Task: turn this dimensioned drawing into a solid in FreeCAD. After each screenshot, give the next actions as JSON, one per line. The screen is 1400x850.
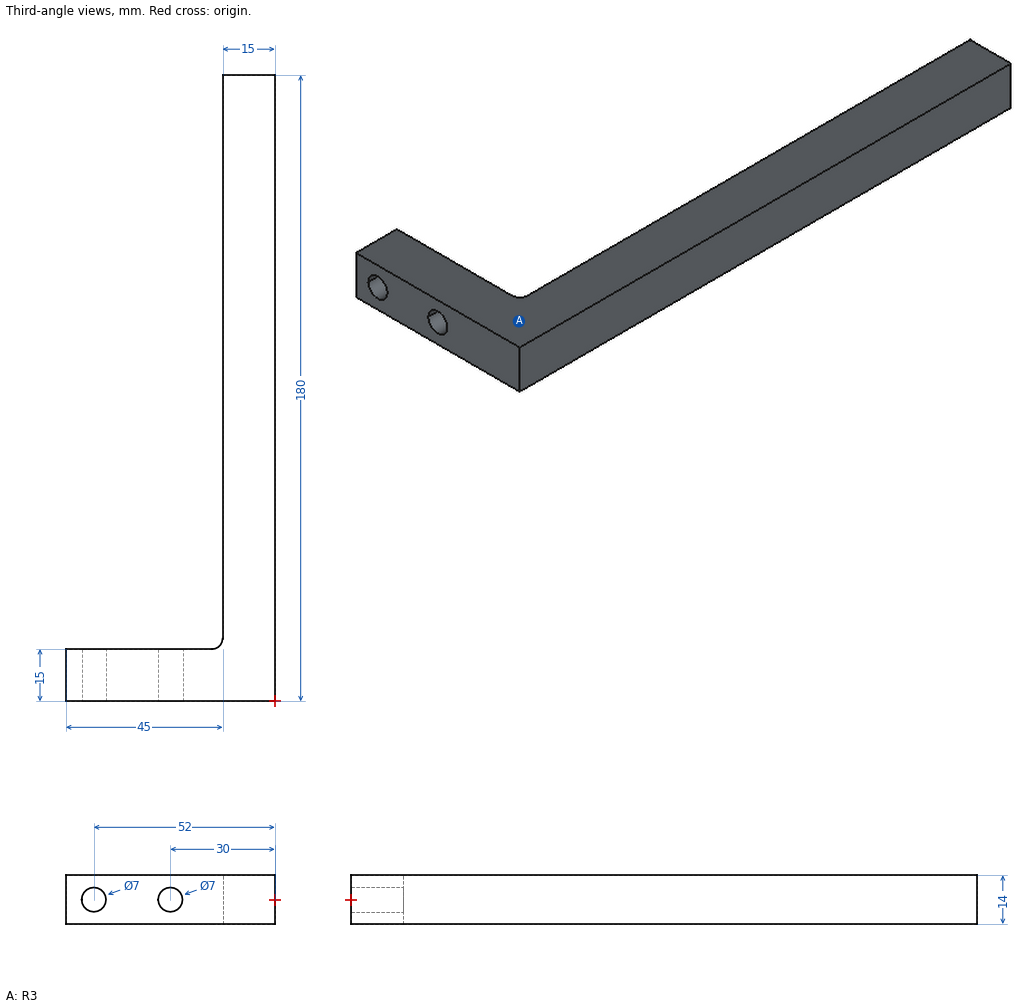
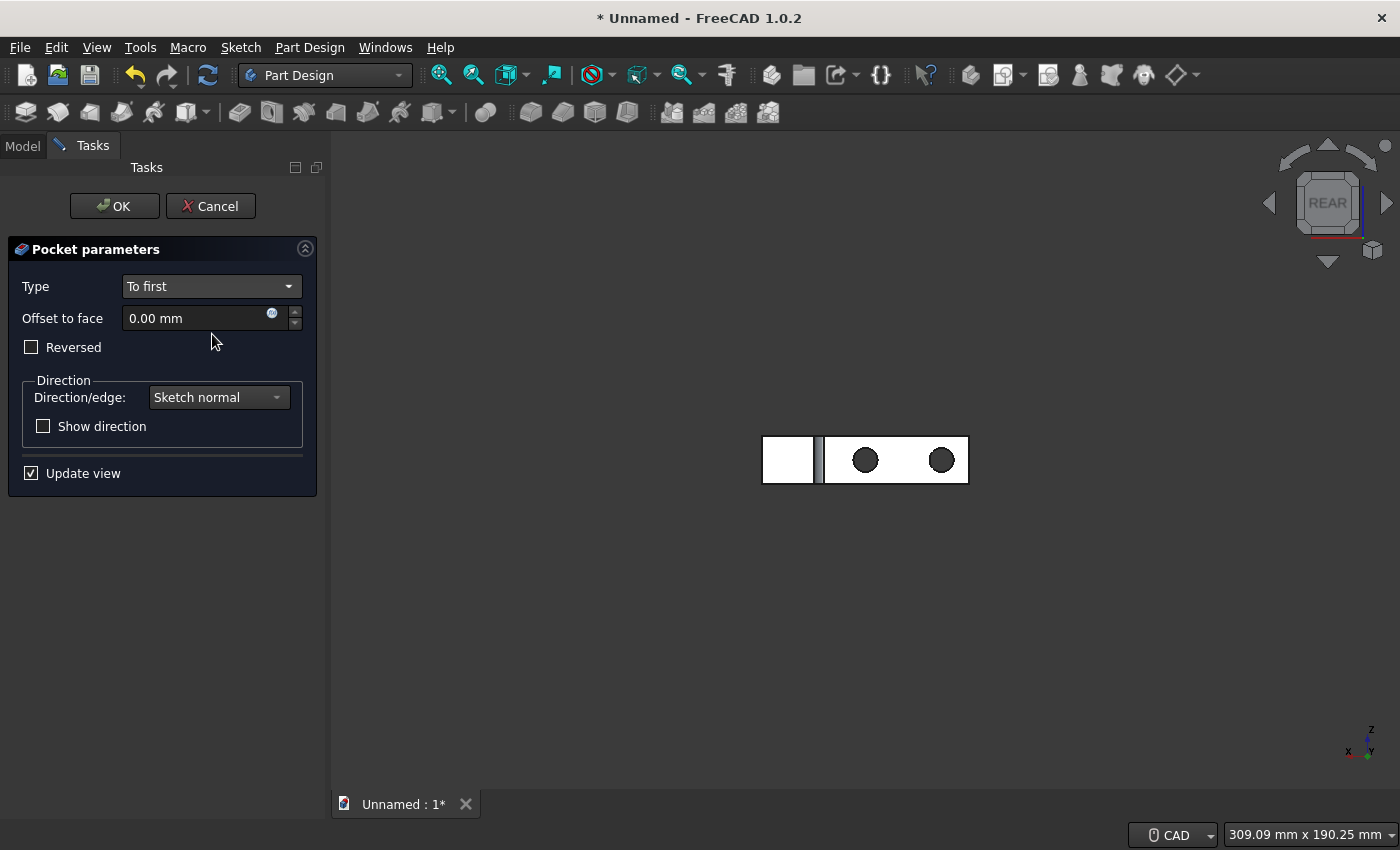
{"action": "left_click", "coordinate": [115, 206]}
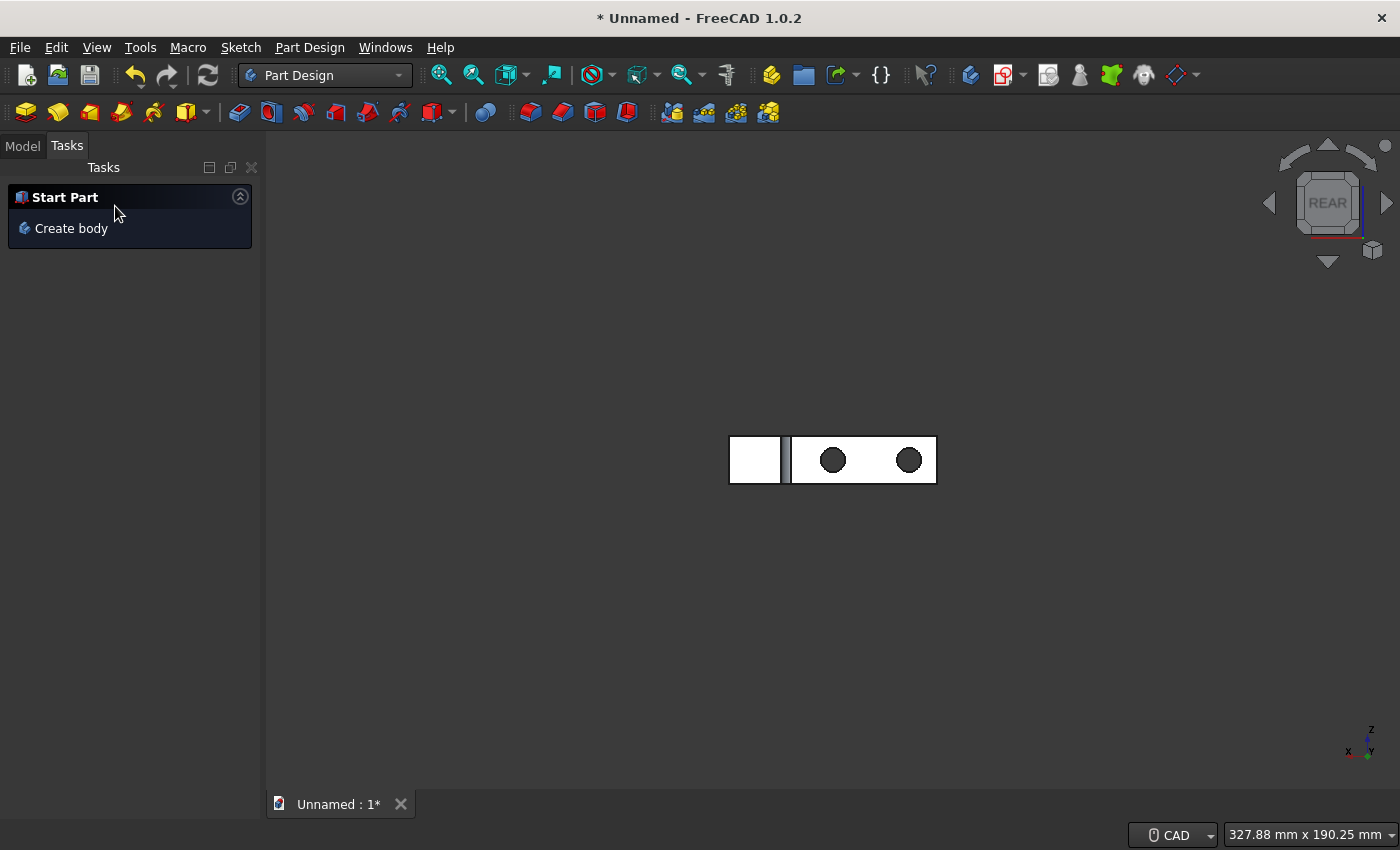
{"action": "key", "text": "0"}